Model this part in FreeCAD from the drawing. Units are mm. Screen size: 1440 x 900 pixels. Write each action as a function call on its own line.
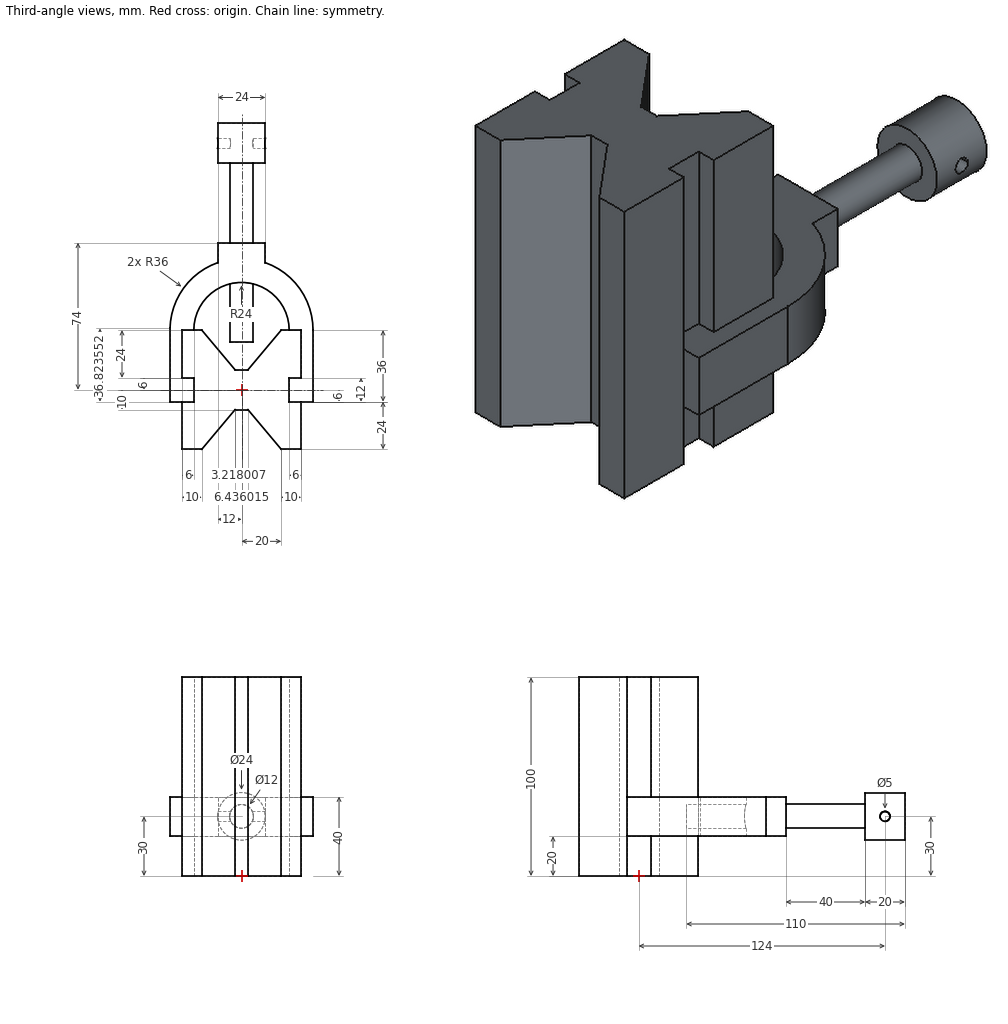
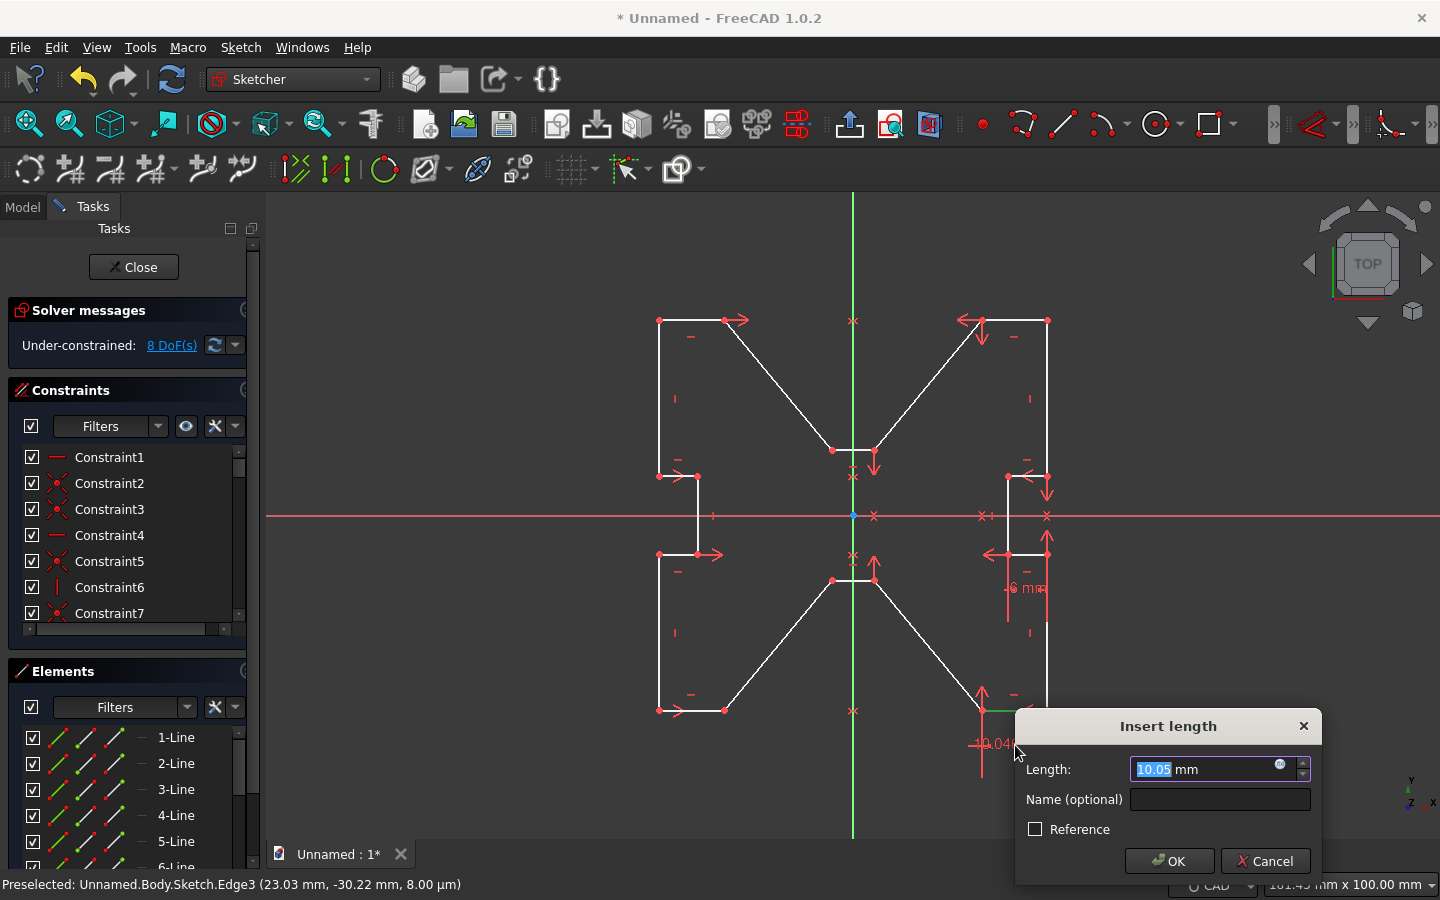
text(10)
key(Return)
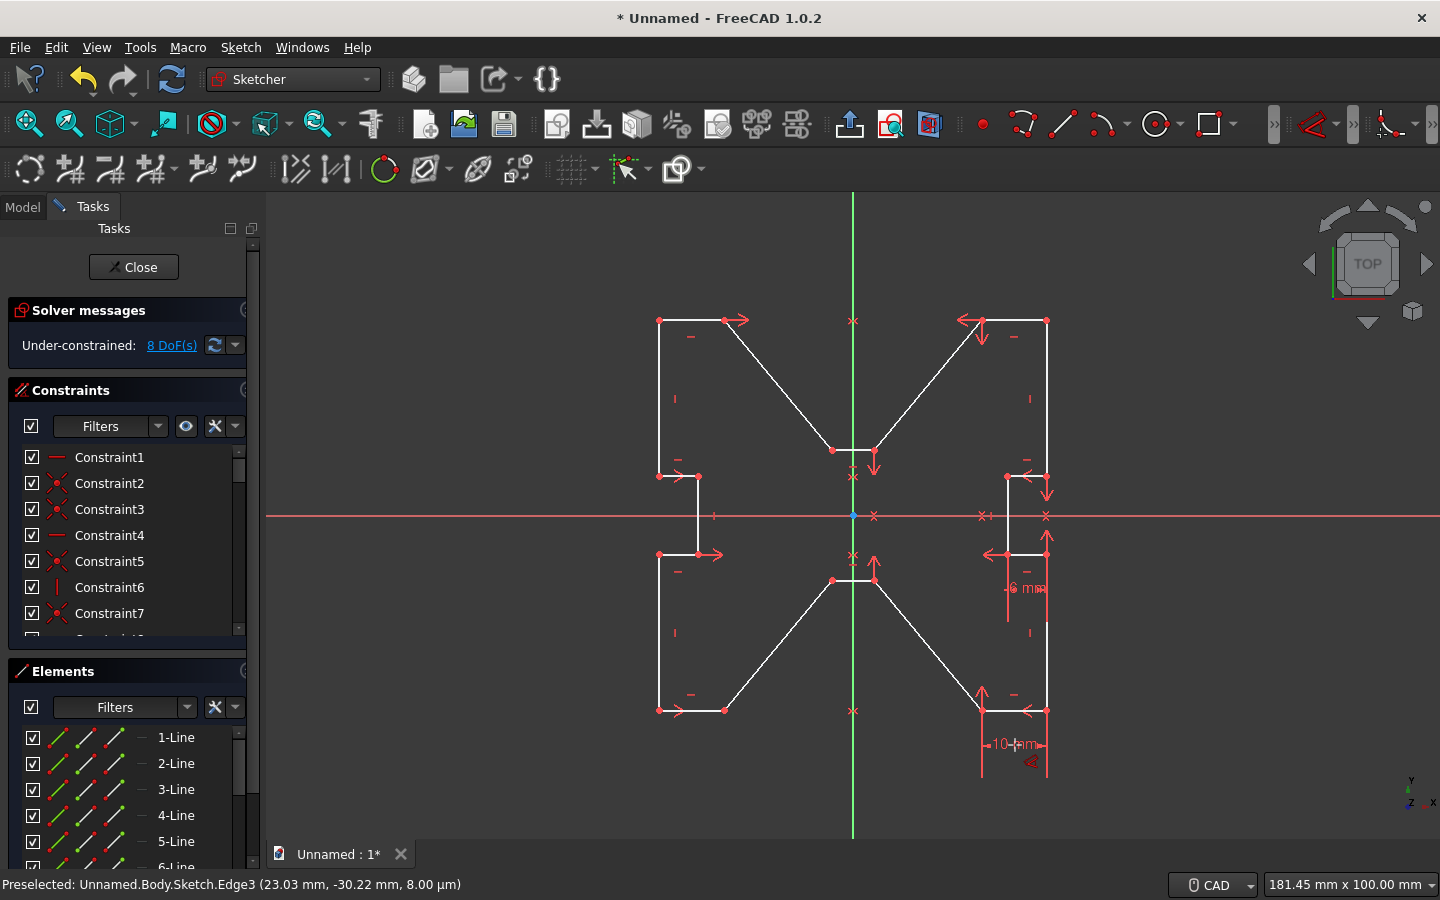
click(1047, 664)
click(1081, 633)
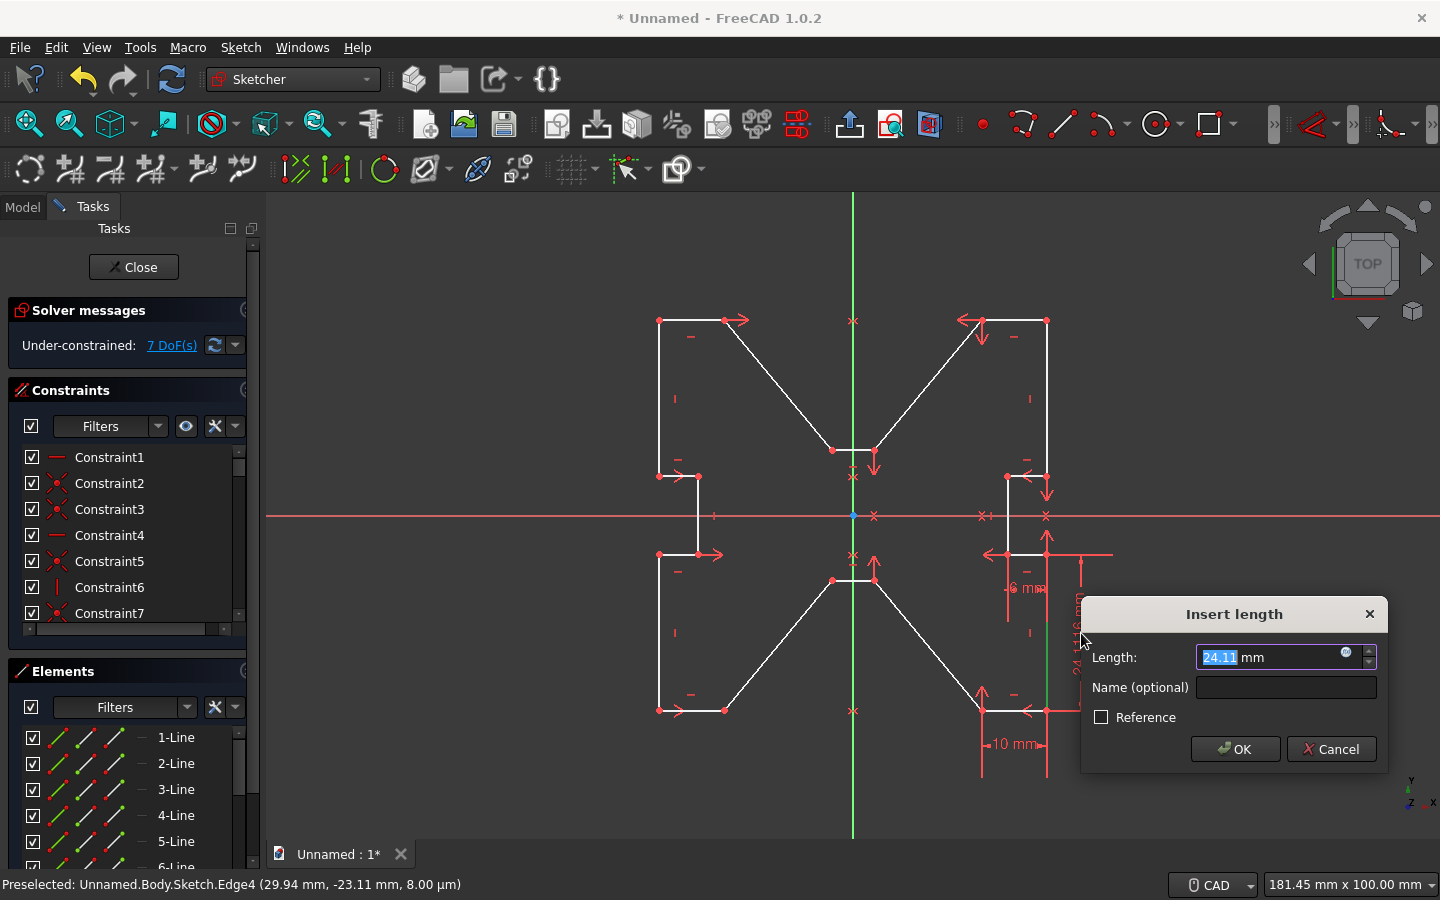
text(24)
key(Return)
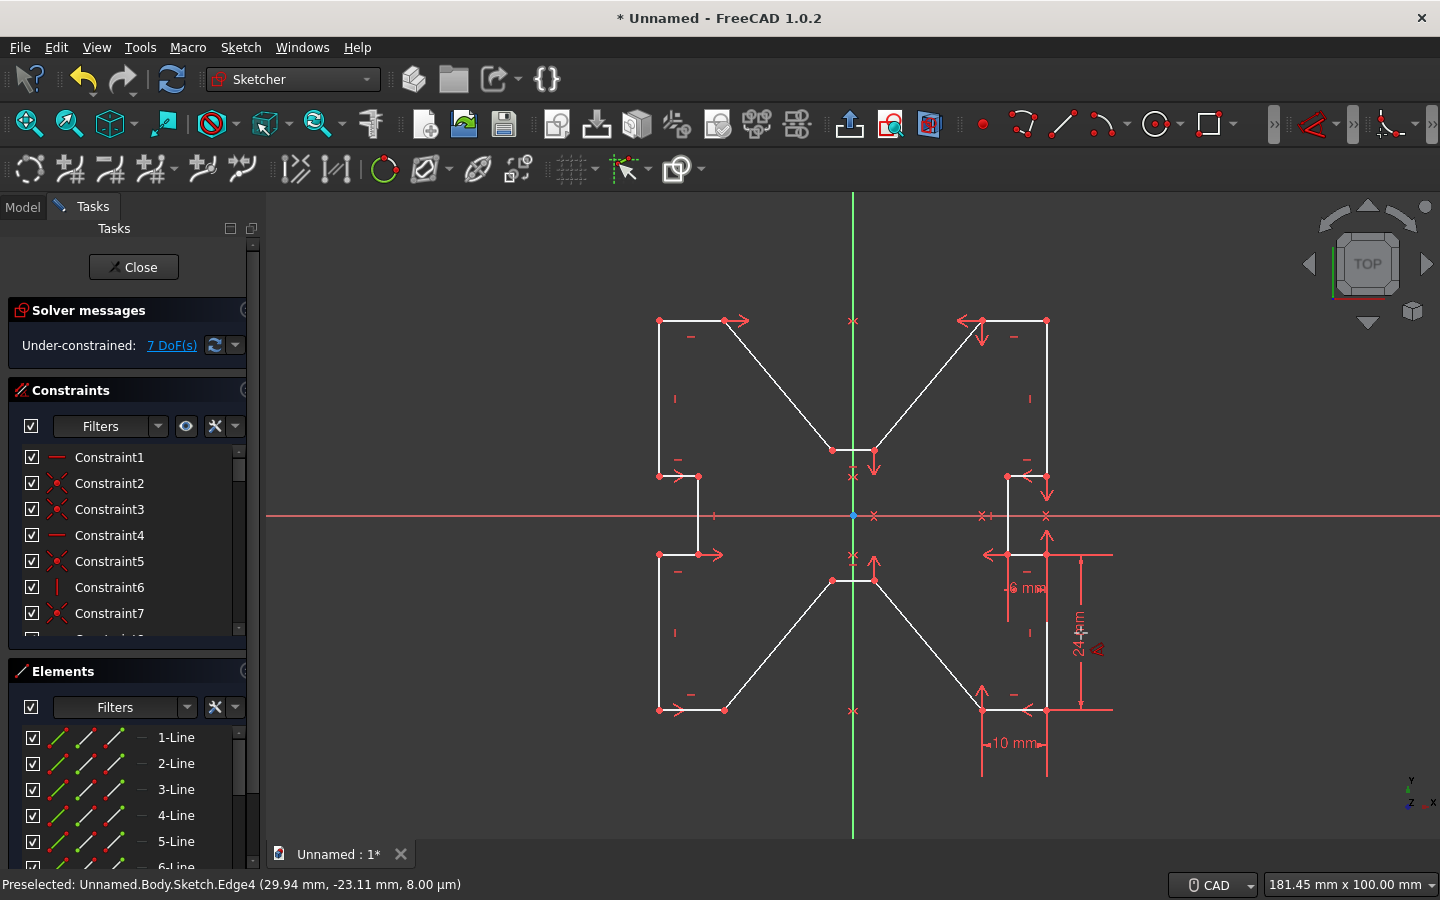
click(1008, 531)
click(1042, 497)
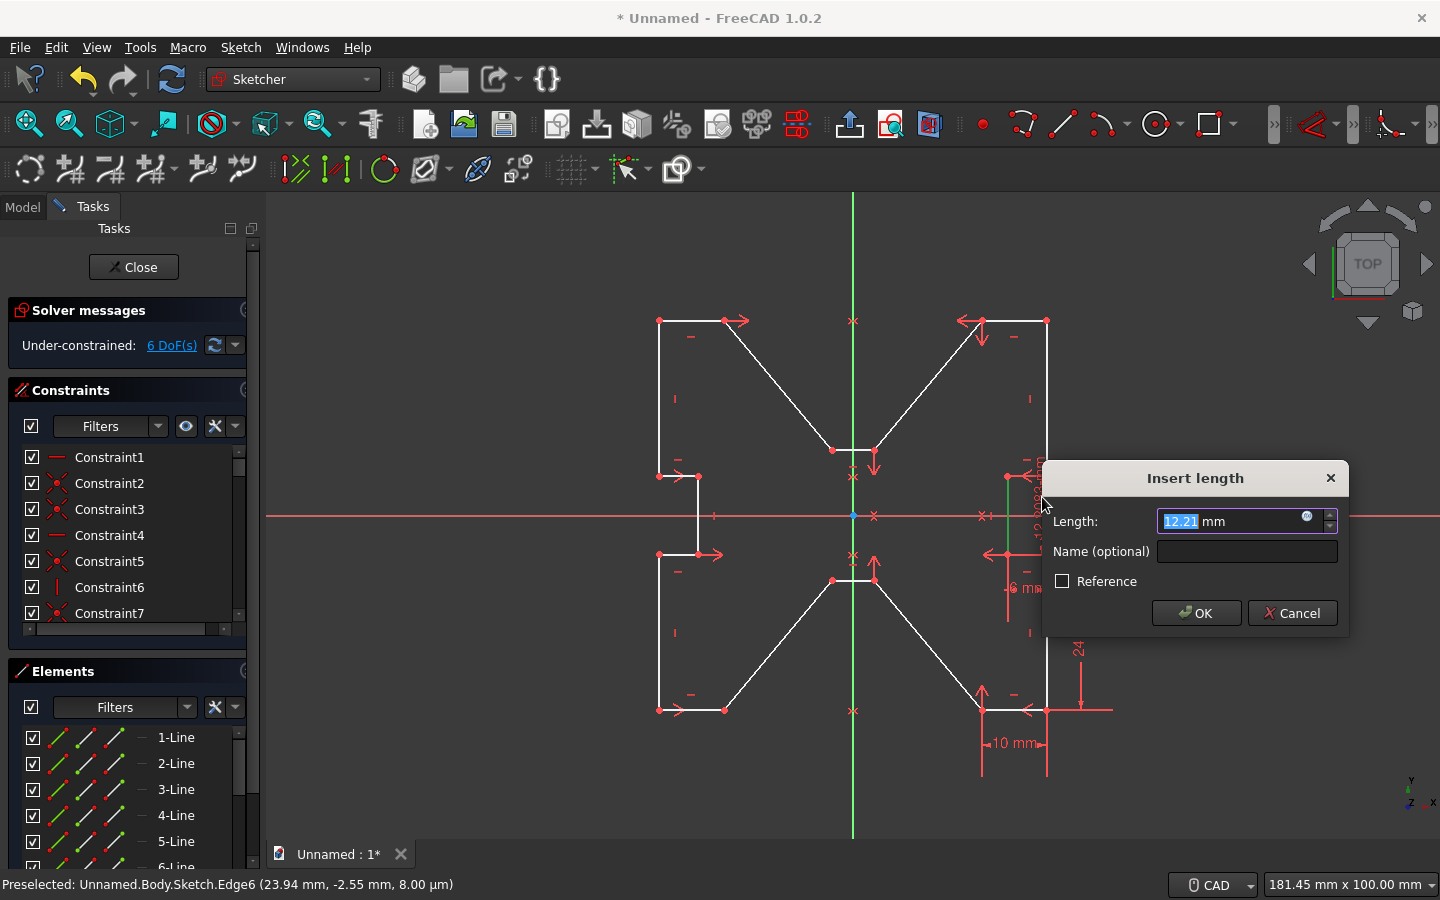
text(12)
key(Return)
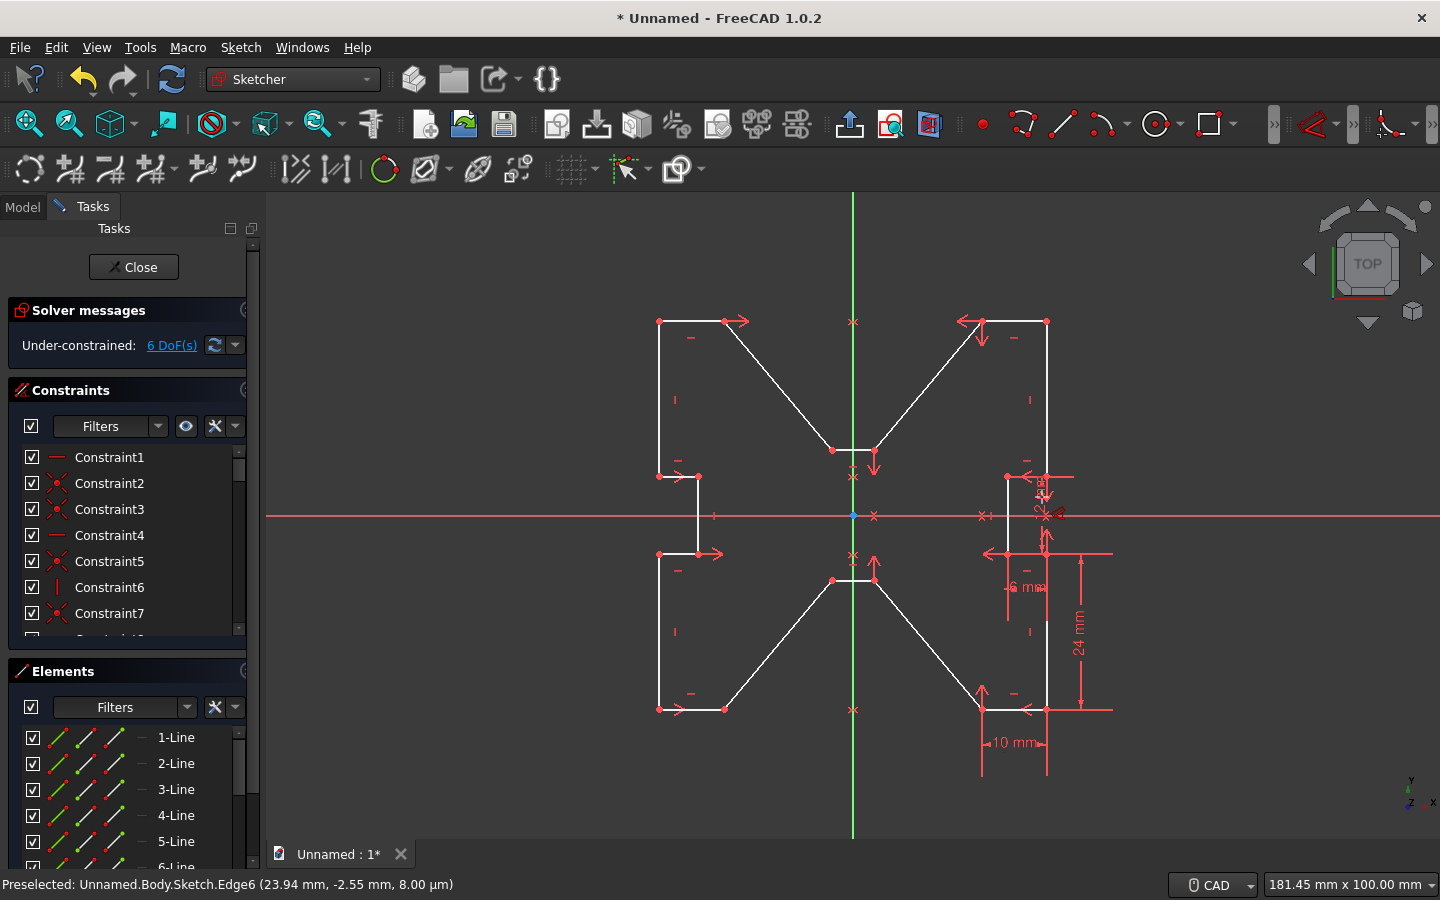
click(679, 710)
click(692, 744)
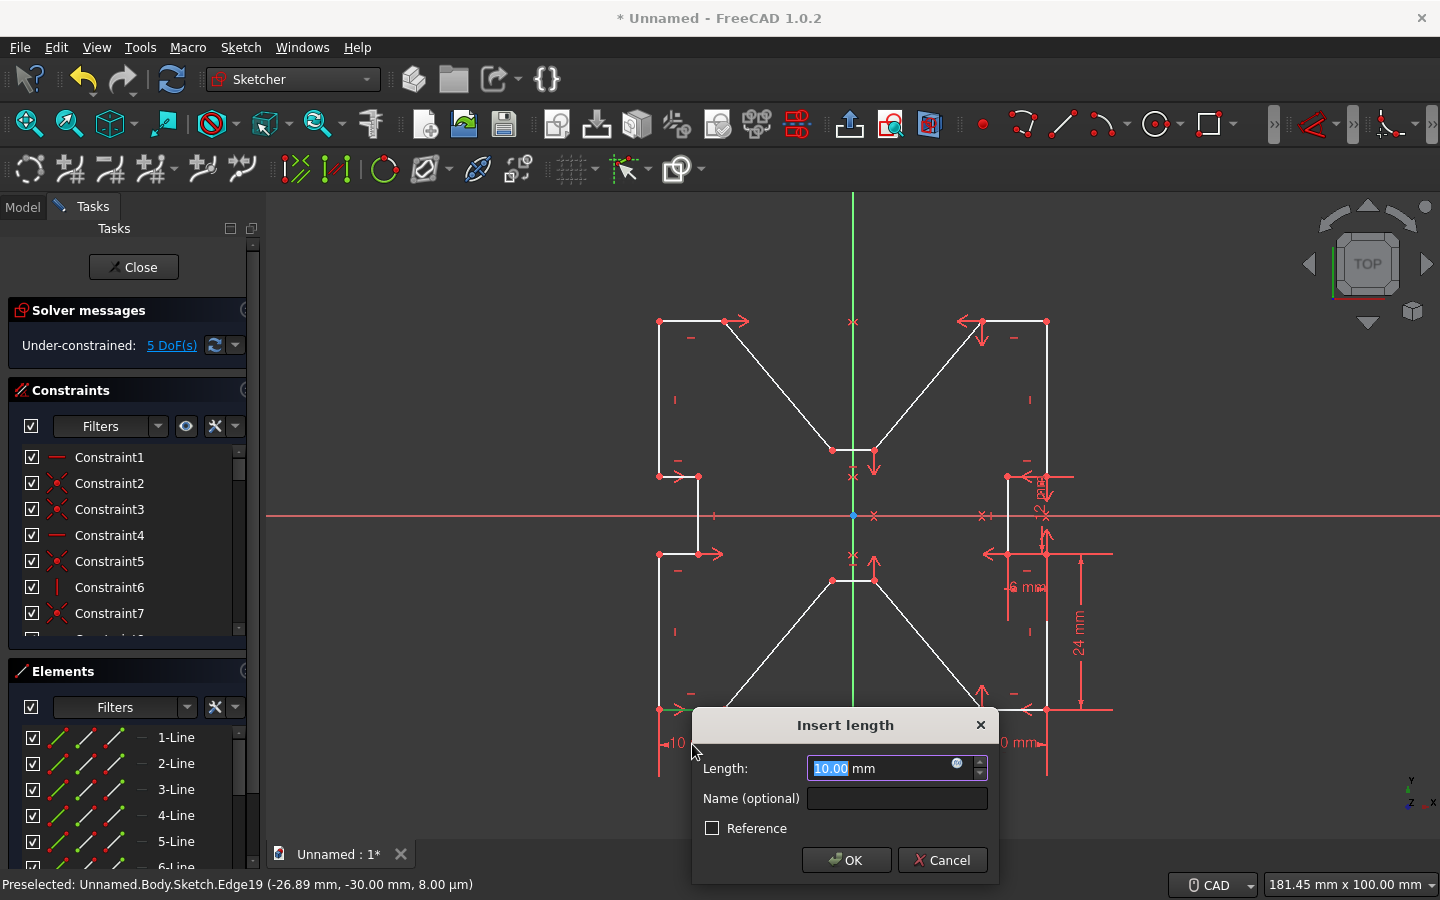
text(10)
key(Return)